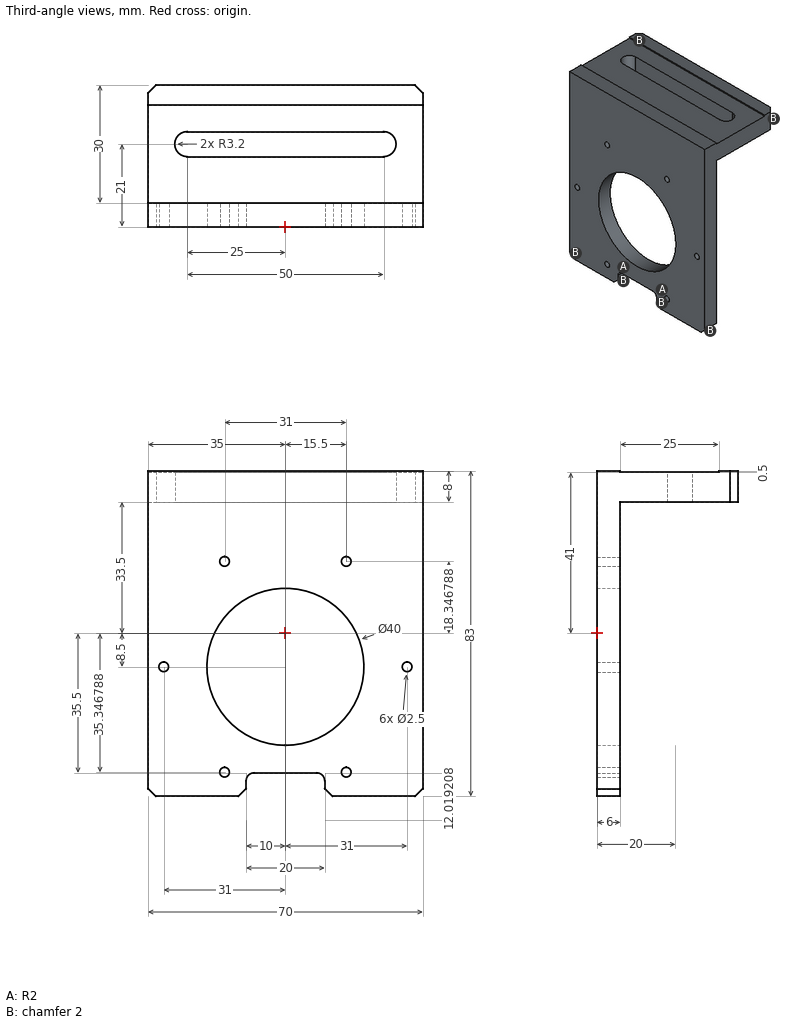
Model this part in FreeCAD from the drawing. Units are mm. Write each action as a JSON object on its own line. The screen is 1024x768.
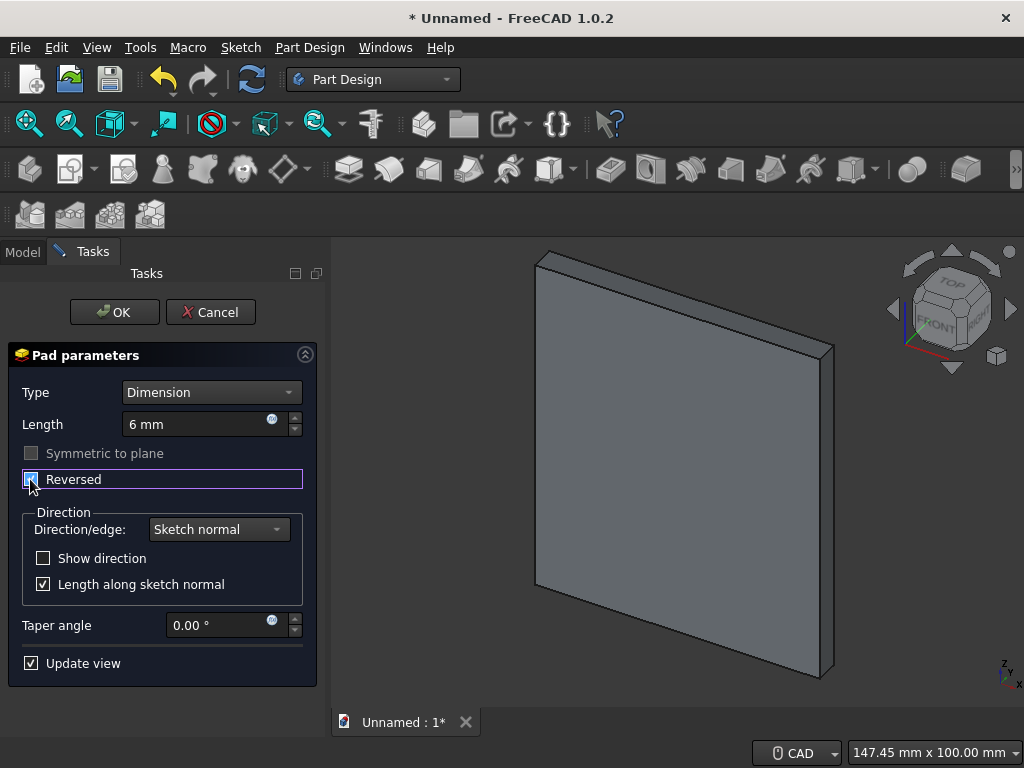
{"action": "left_click", "coordinate": [115, 312]}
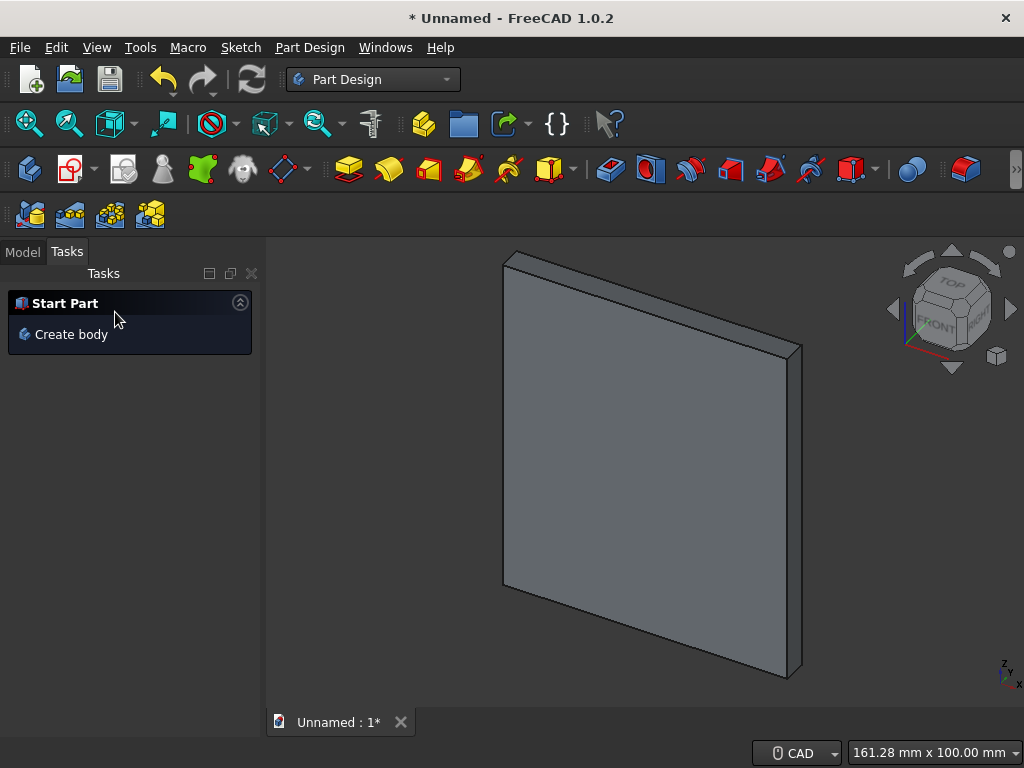
{"action": "key", "text": "4"}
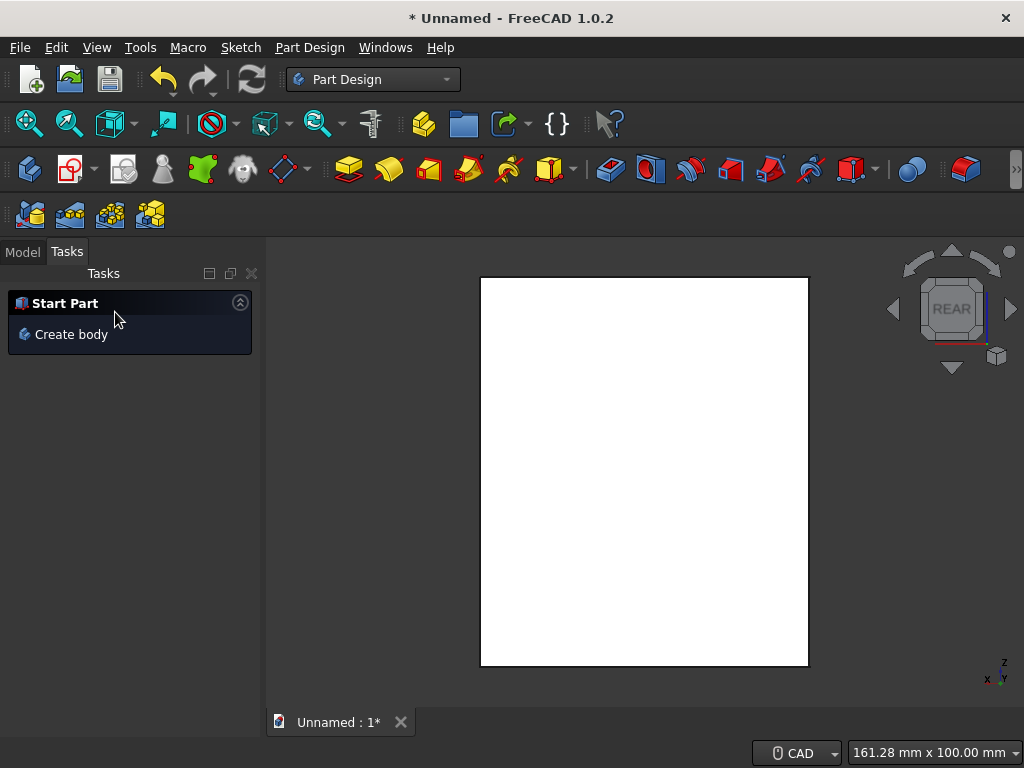
{"action": "left_click", "coordinate": [645, 471]}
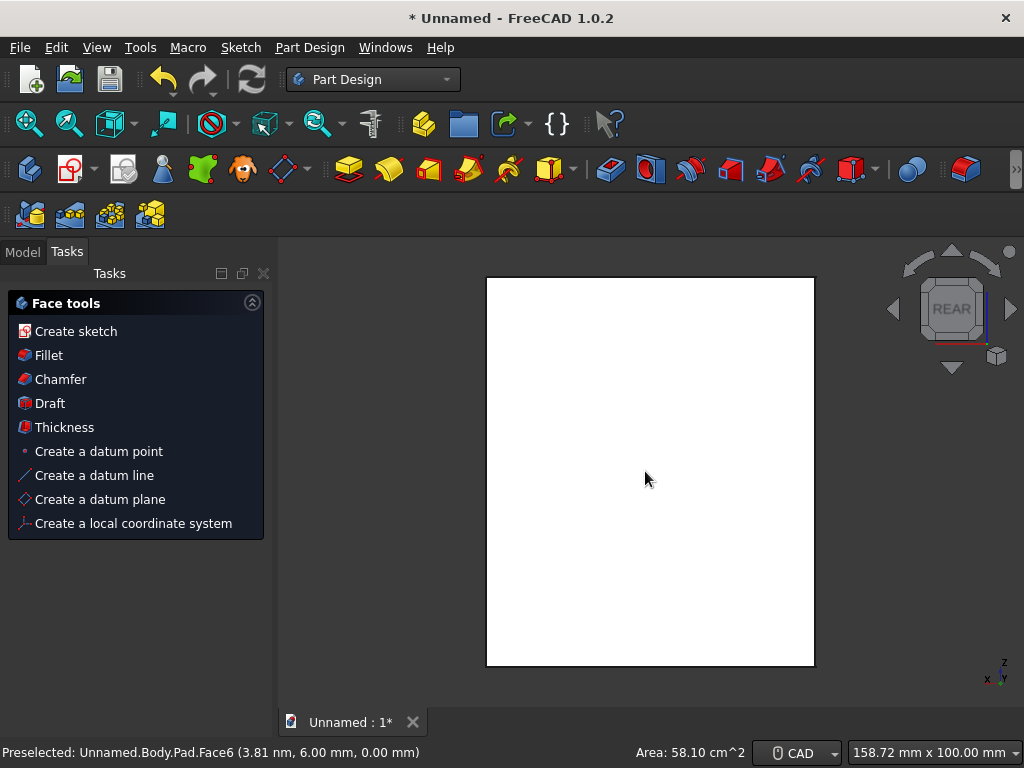
{"action": "left_click", "coordinate": [70, 170]}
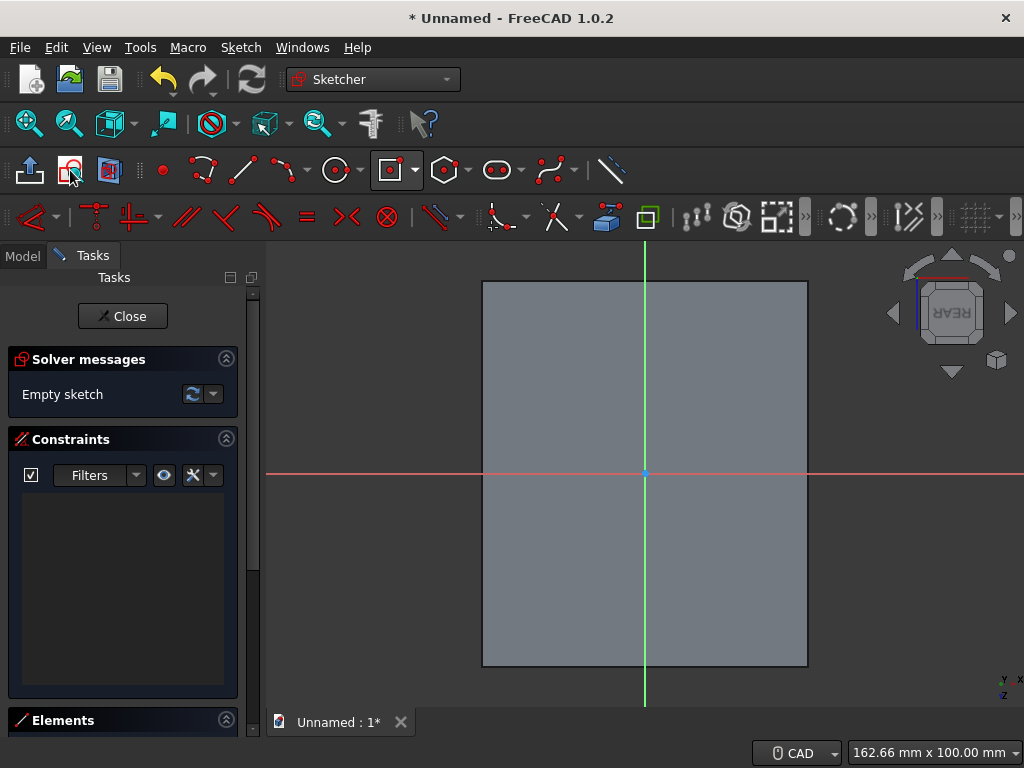
{"action": "scroll", "coordinate": [294, 269], "scroll_direction": "down", "scroll_amount": 1}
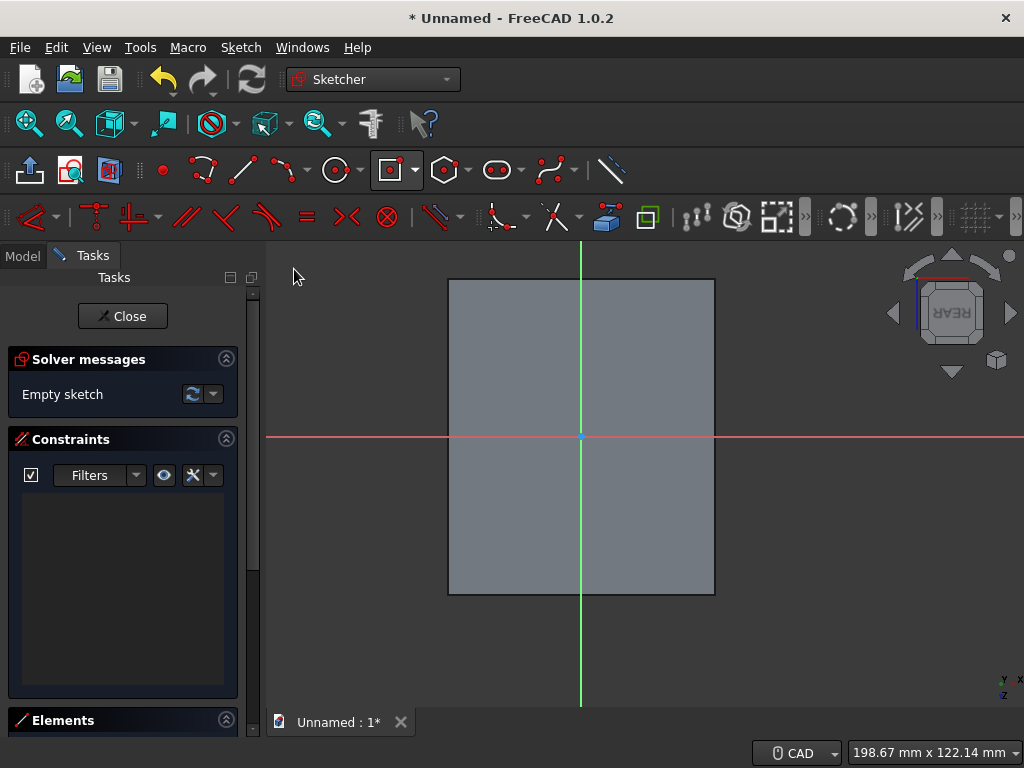
{"action": "scroll", "coordinate": [591, 601], "scroll_direction": "up", "scroll_amount": 2}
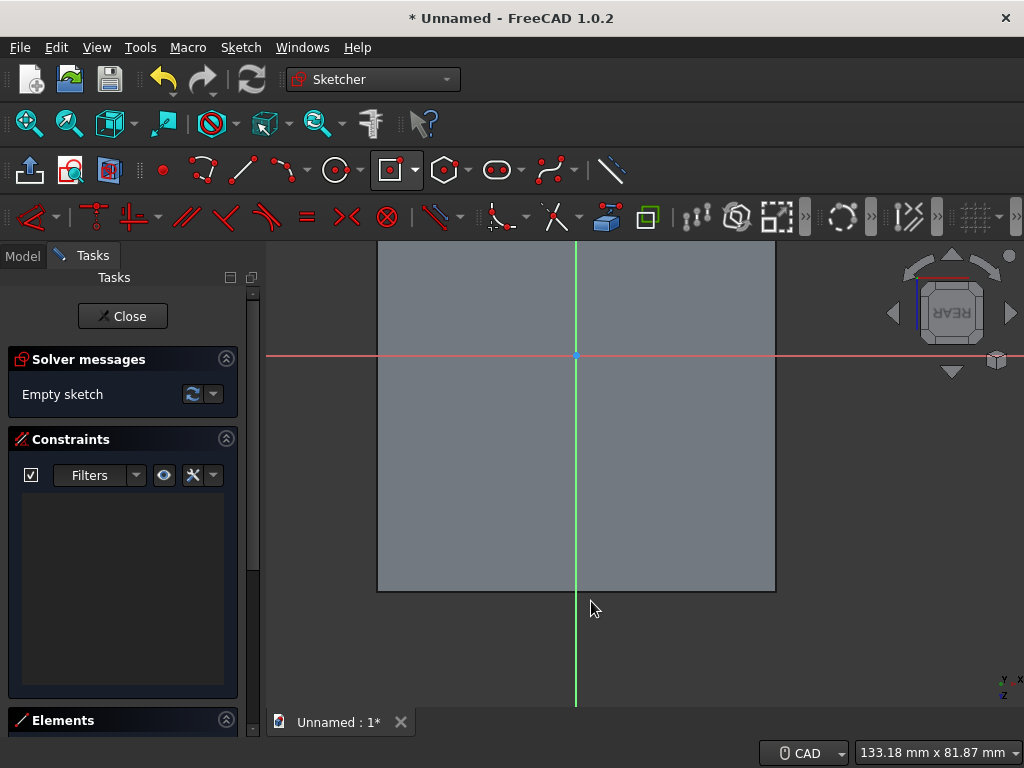
{"action": "key", "text": "g r"}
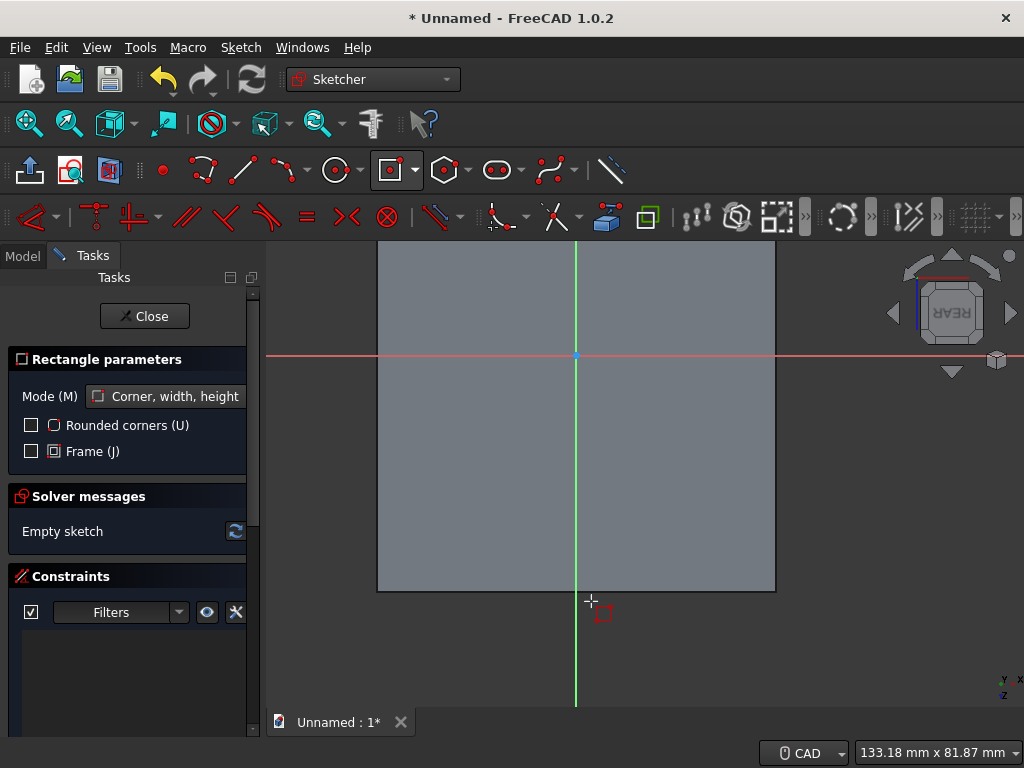
{"action": "left_click", "coordinate": [377, 546]}
{"action": "mouse_move", "coordinate": [776, 592]}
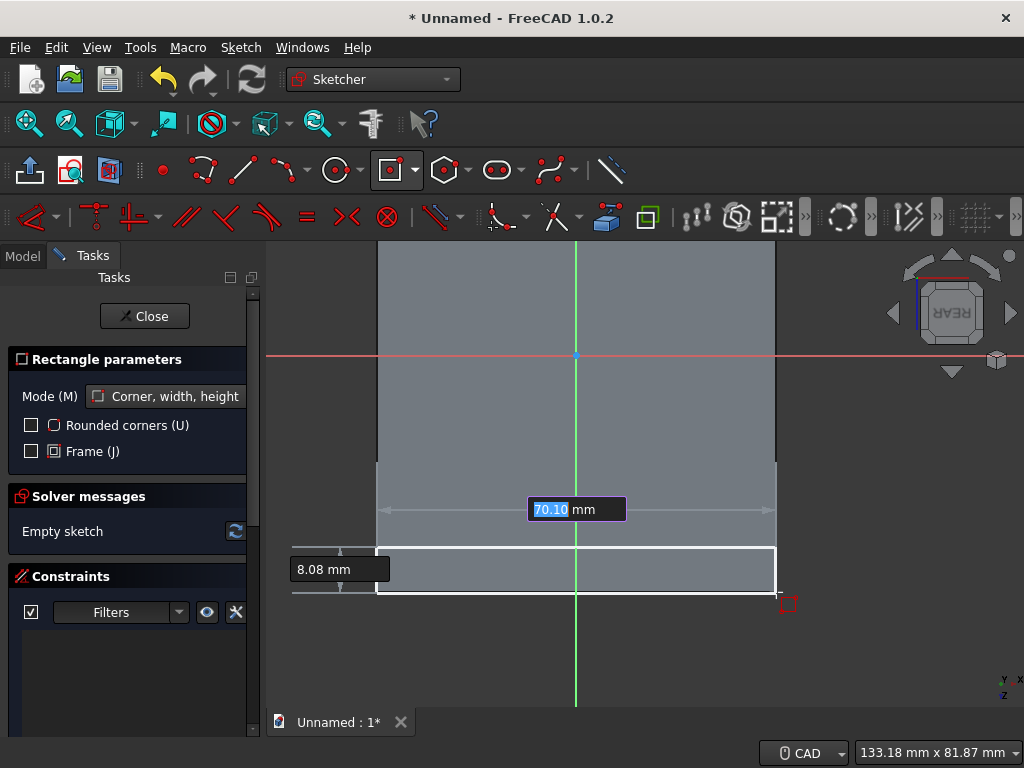
{"action": "type", "text": "70"}
{"action": "key", "text": "Tab"}
{"action": "type", "text": "8"}
{"action": "key", "text": "Return"}
{"action": "key", "text": "Escape"}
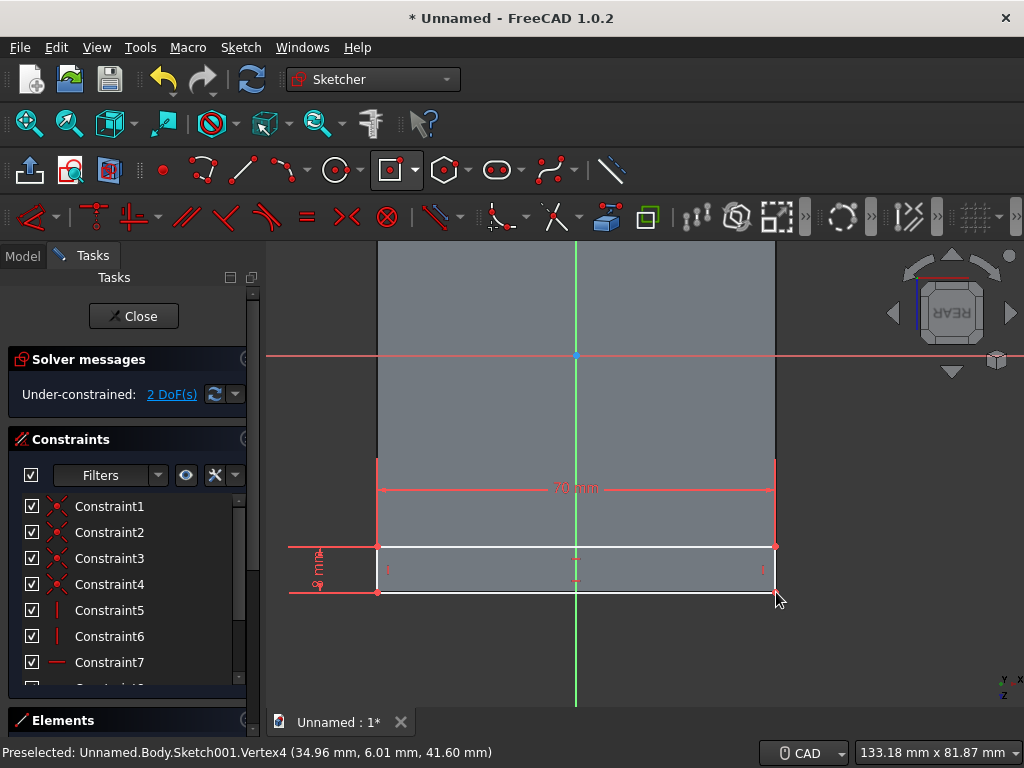
{"action": "left_click", "coordinate": [377, 547]}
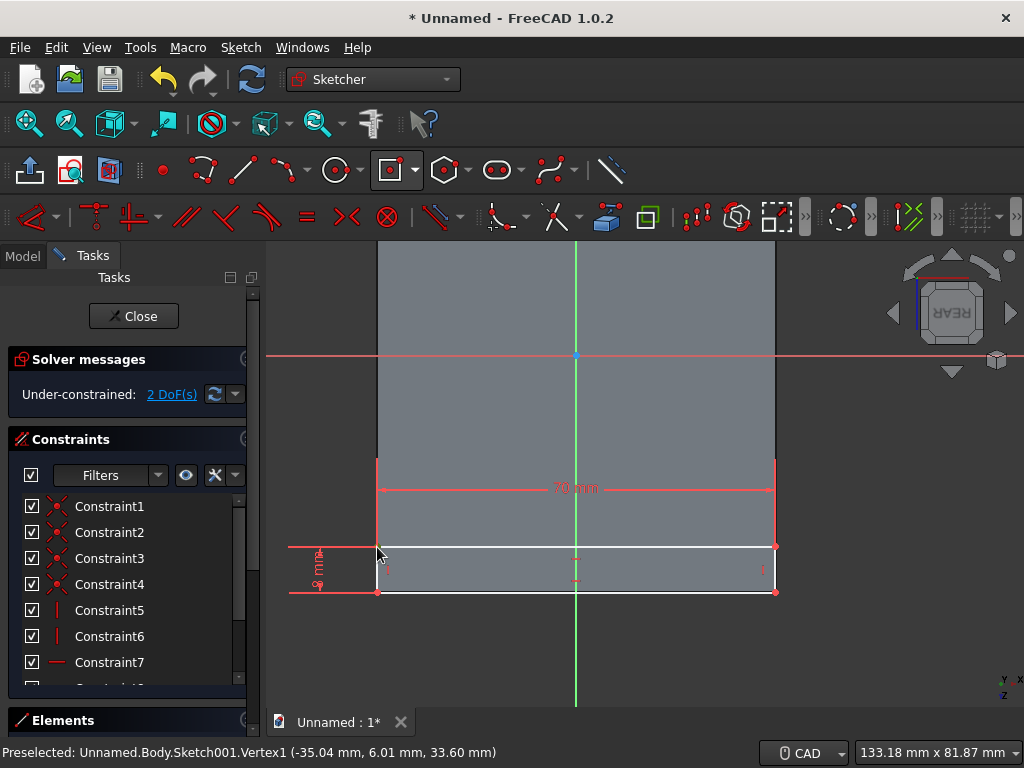
{"action": "left_click", "coordinate": [58, 218]}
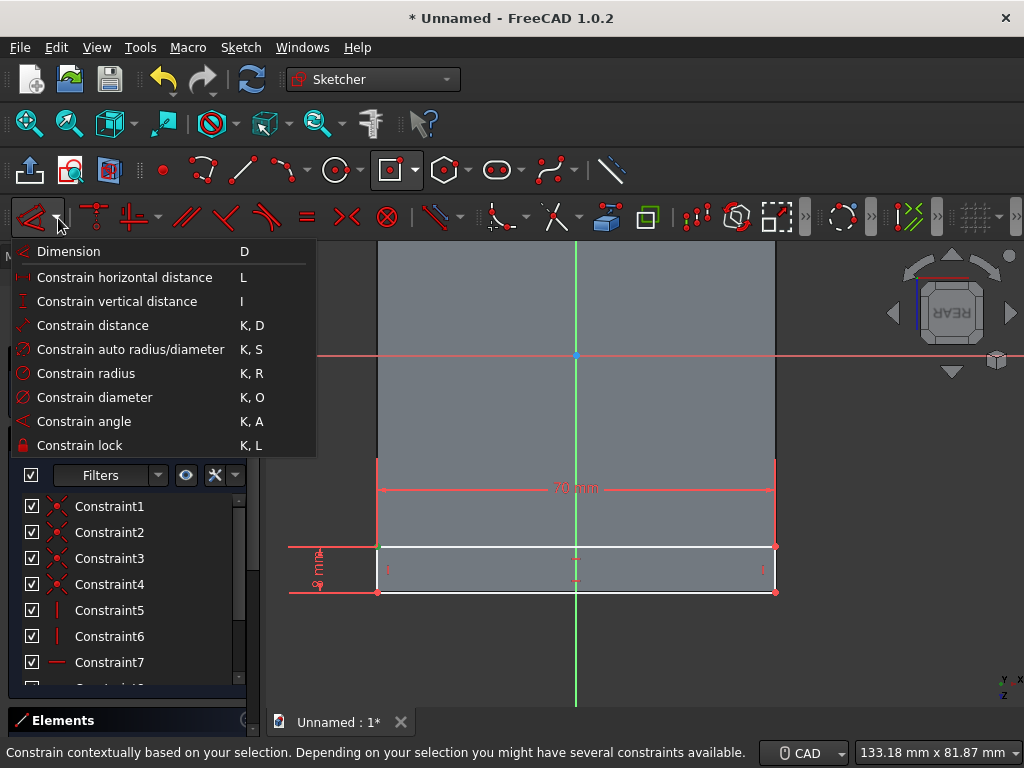
{"action": "left_click", "coordinate": [164, 277]}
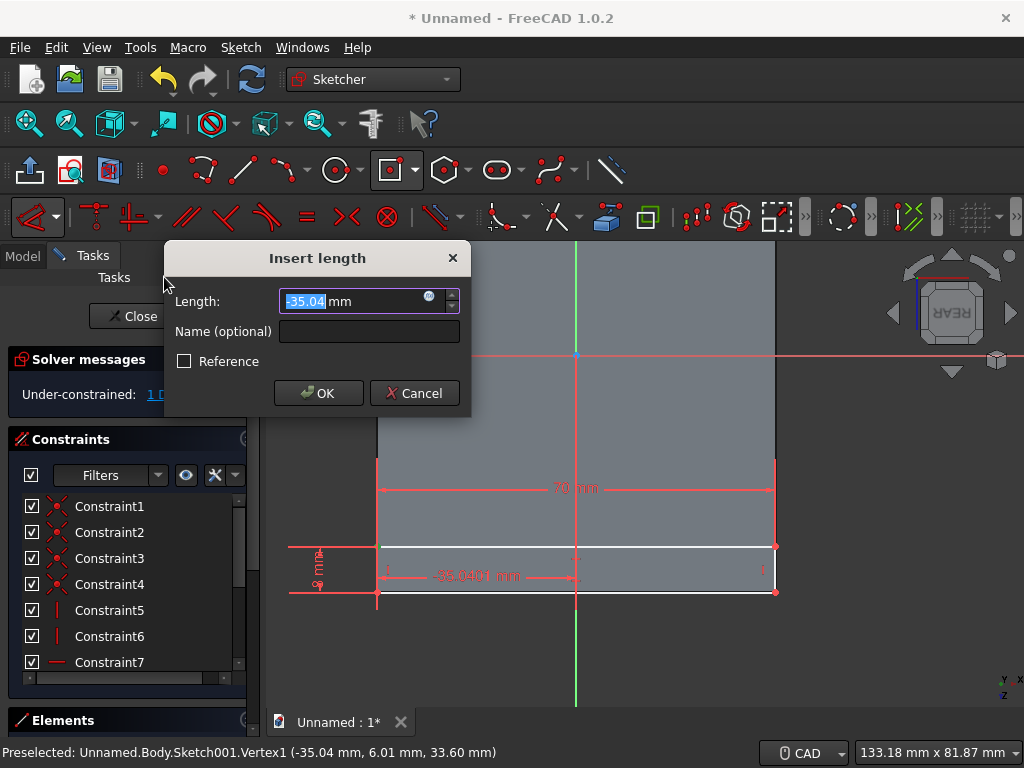
{"action": "type", "text": "-35"}
{"action": "key", "text": "Return"}